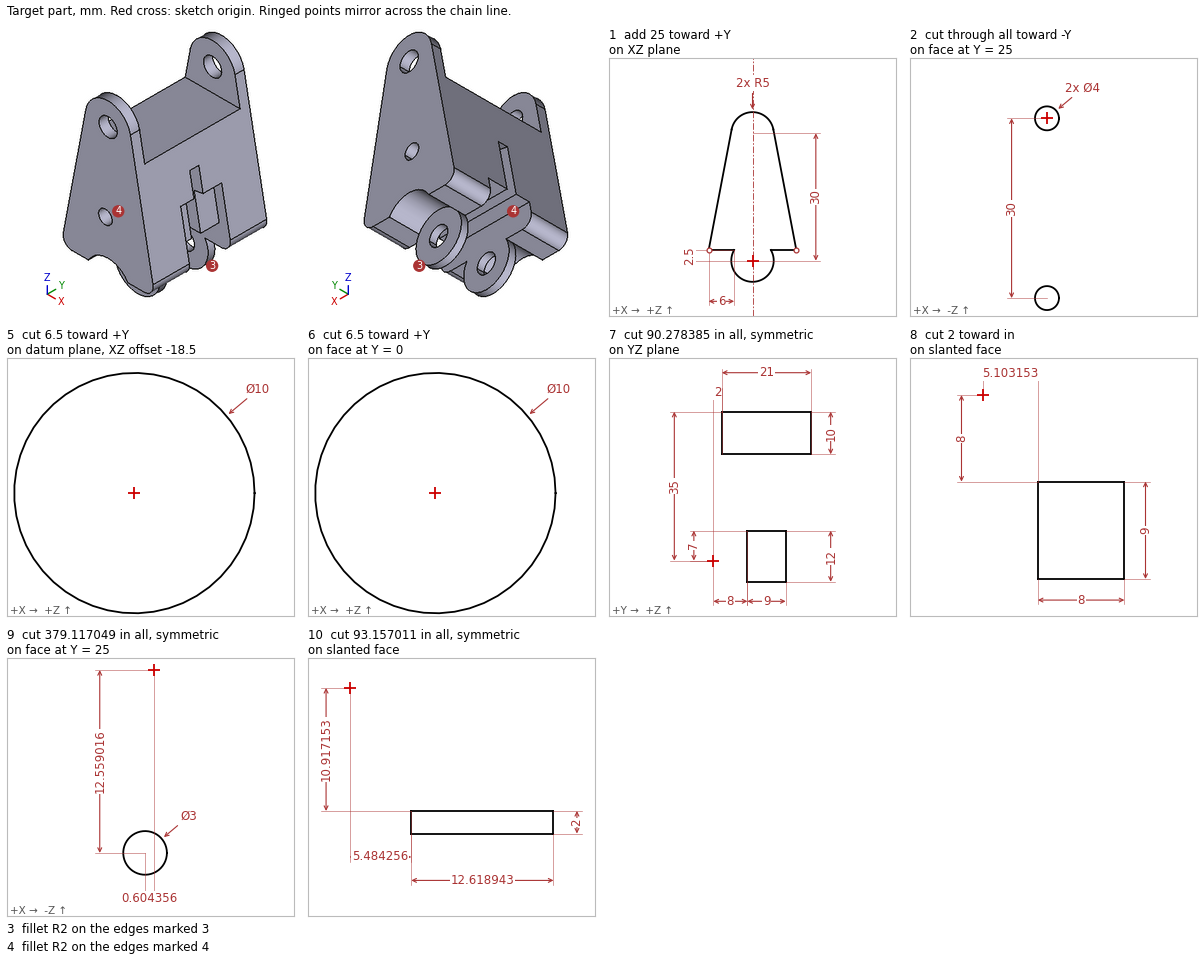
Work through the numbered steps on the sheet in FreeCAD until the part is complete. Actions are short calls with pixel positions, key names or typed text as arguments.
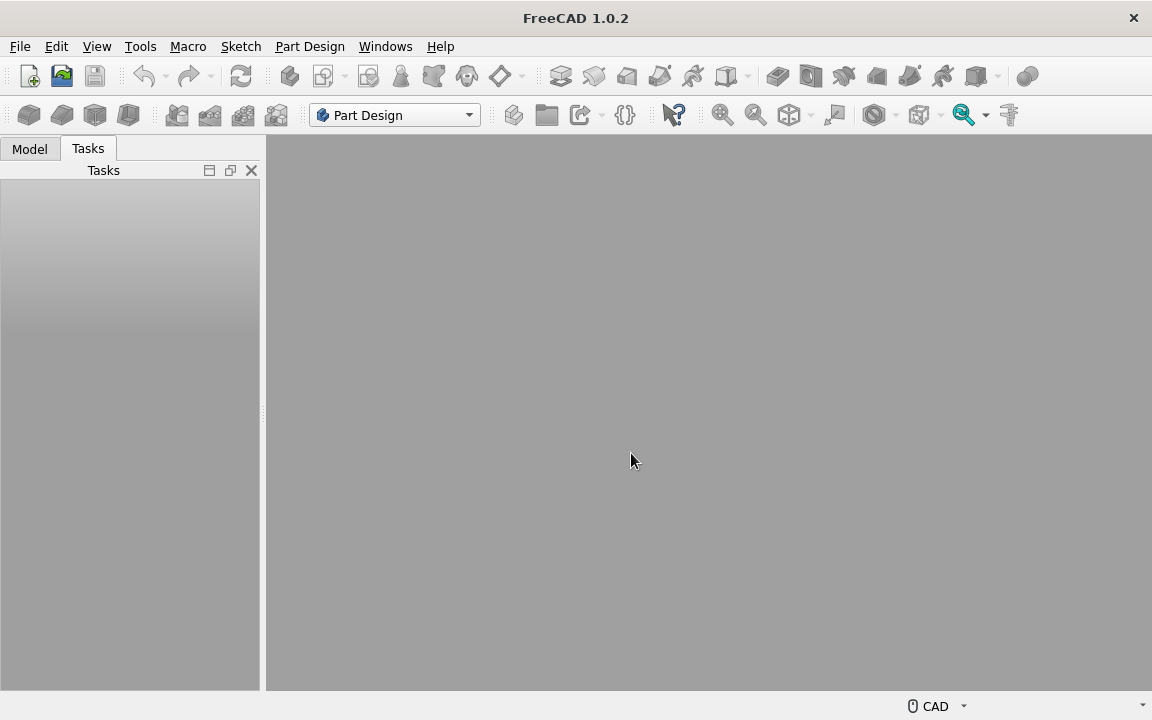
key(ctrl+n)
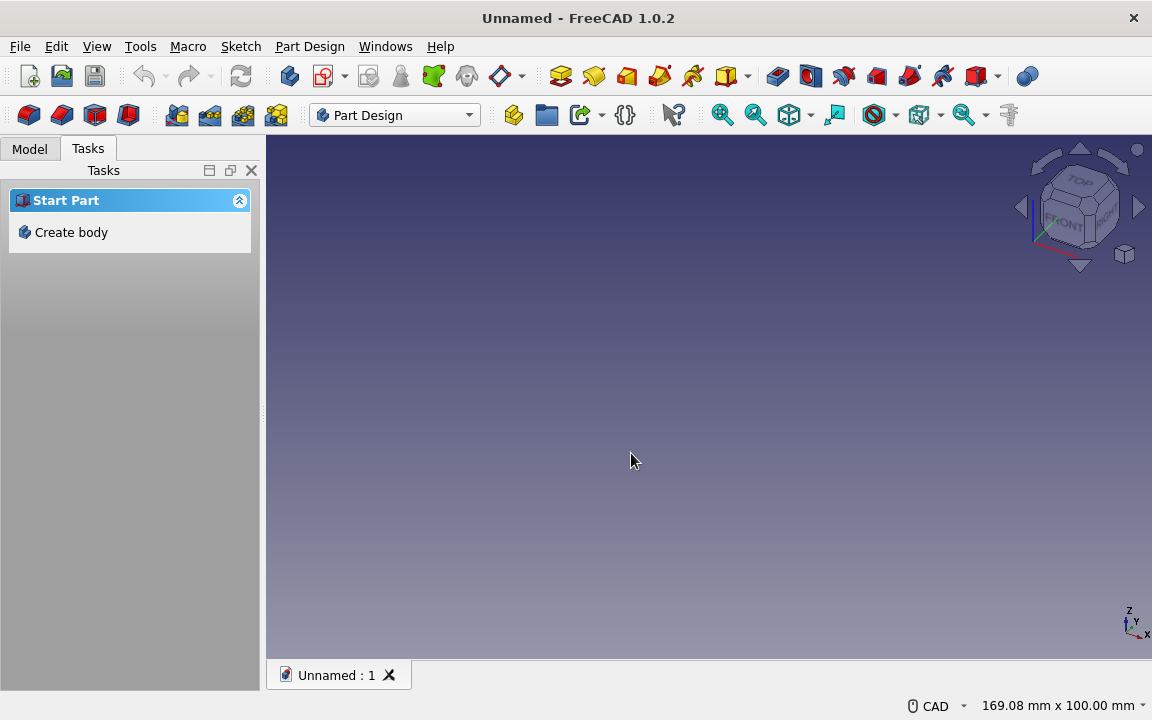
click(322, 76)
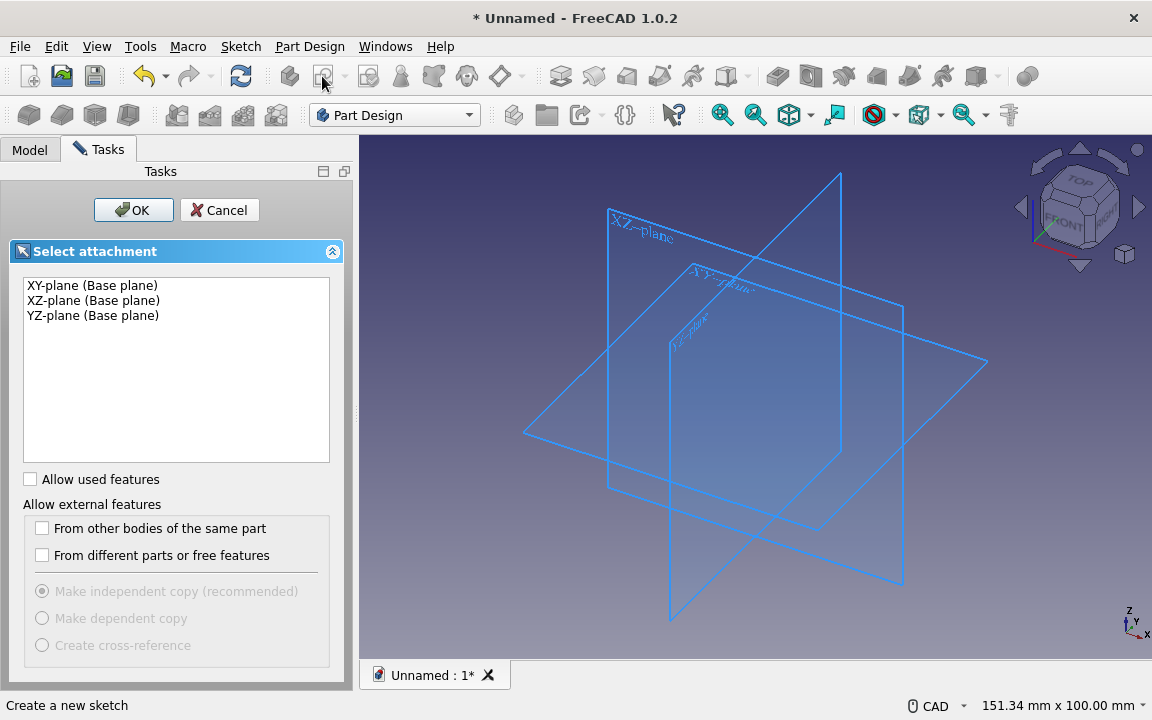
click(84, 300)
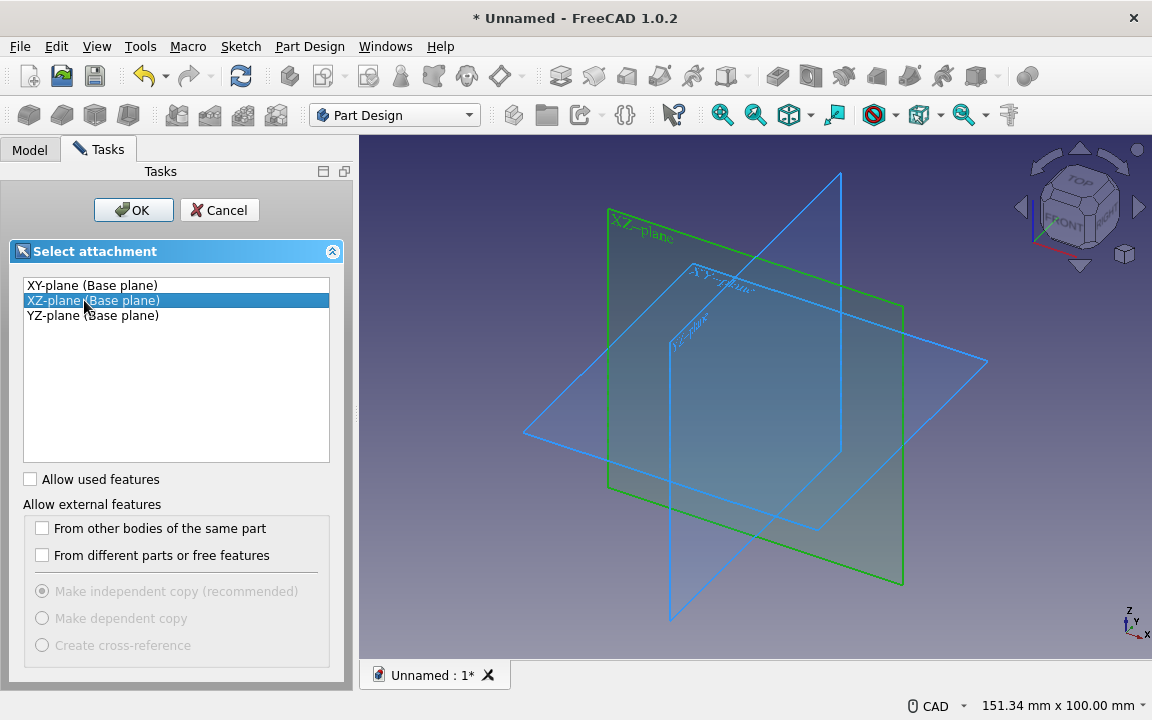
click(134, 210)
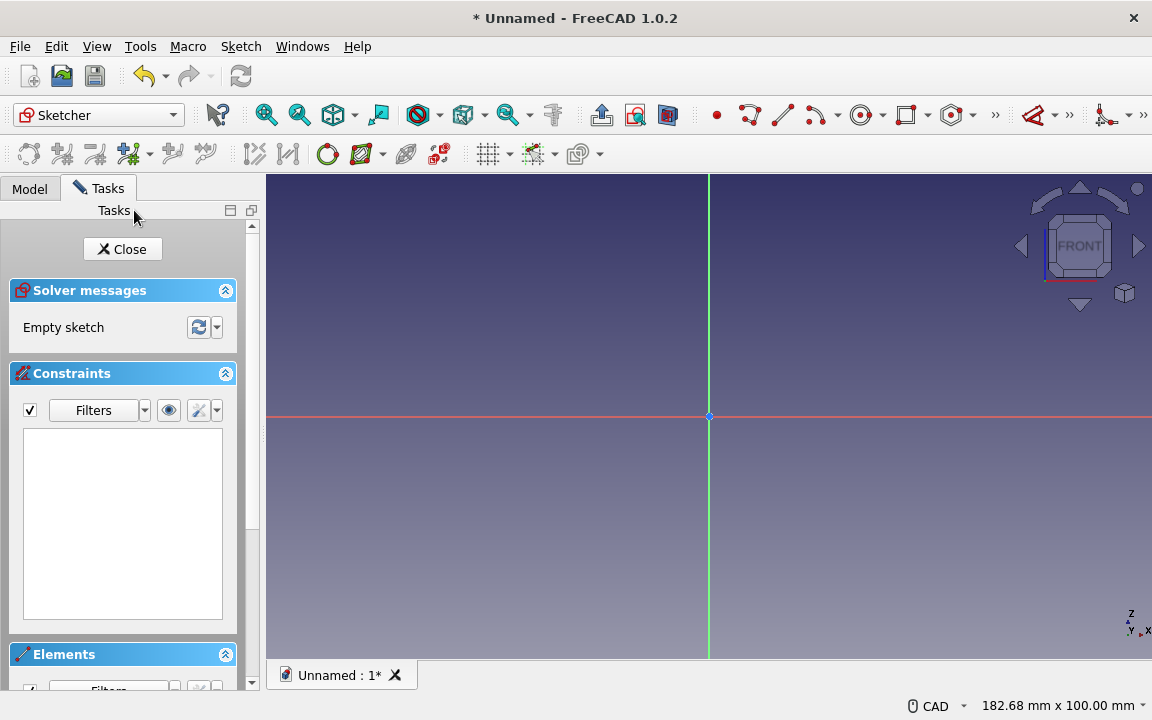
scroll(848, 202, up, 2)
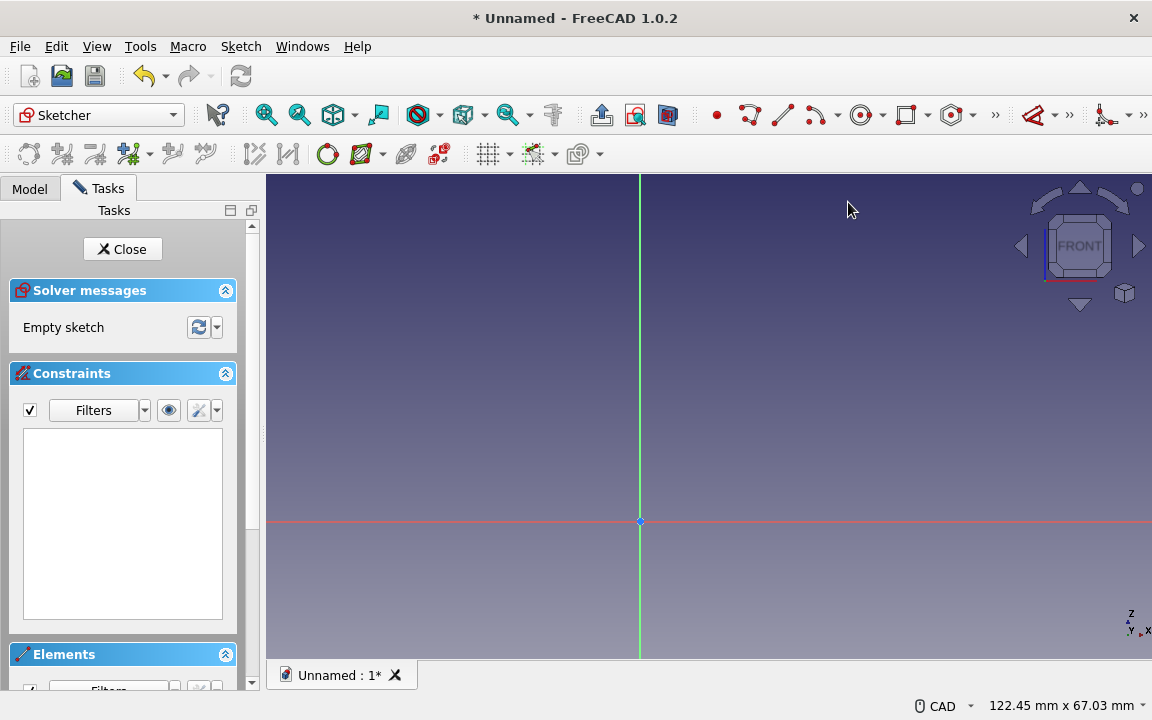
click(750, 116)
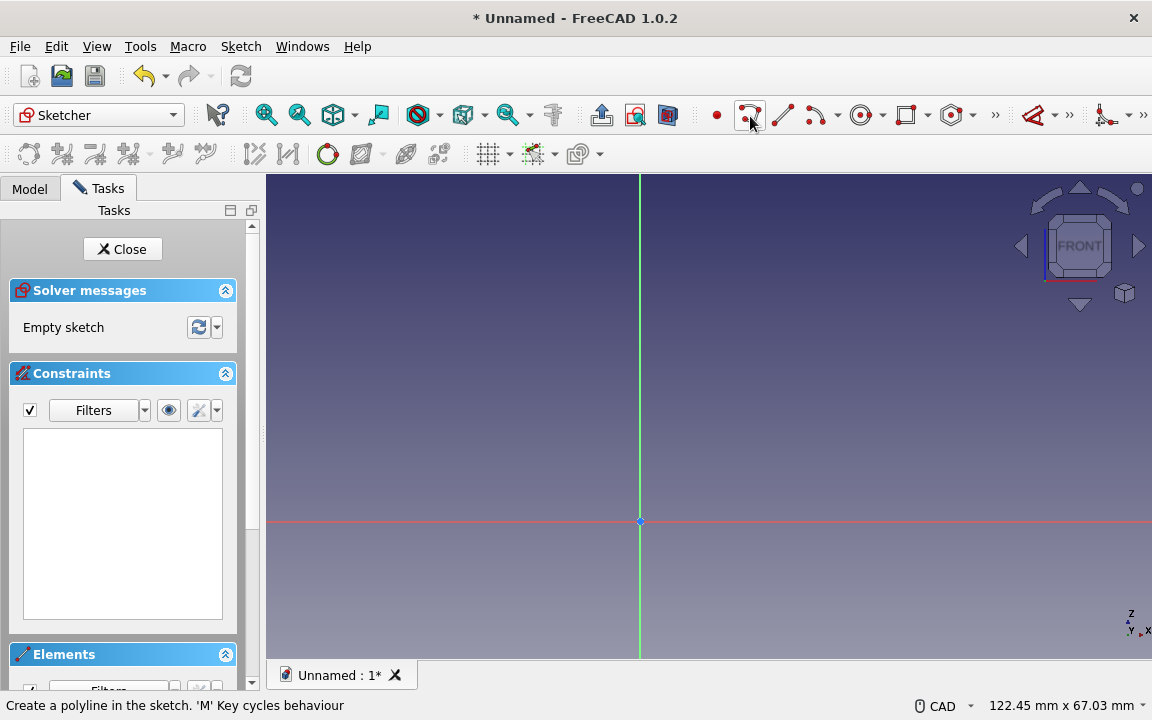
click(609, 504)
click(566, 504)
click(605, 298)
right_click(605, 298)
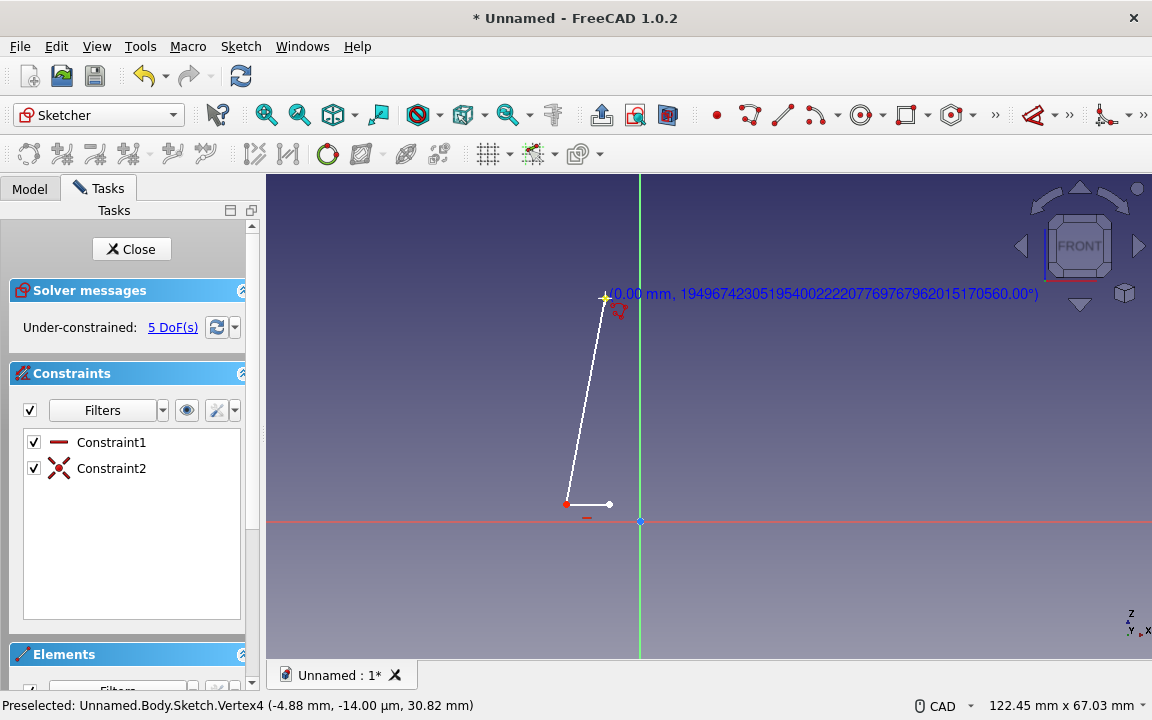
click(676, 298)
click(715, 504)
click(672, 504)
right_click(672, 504)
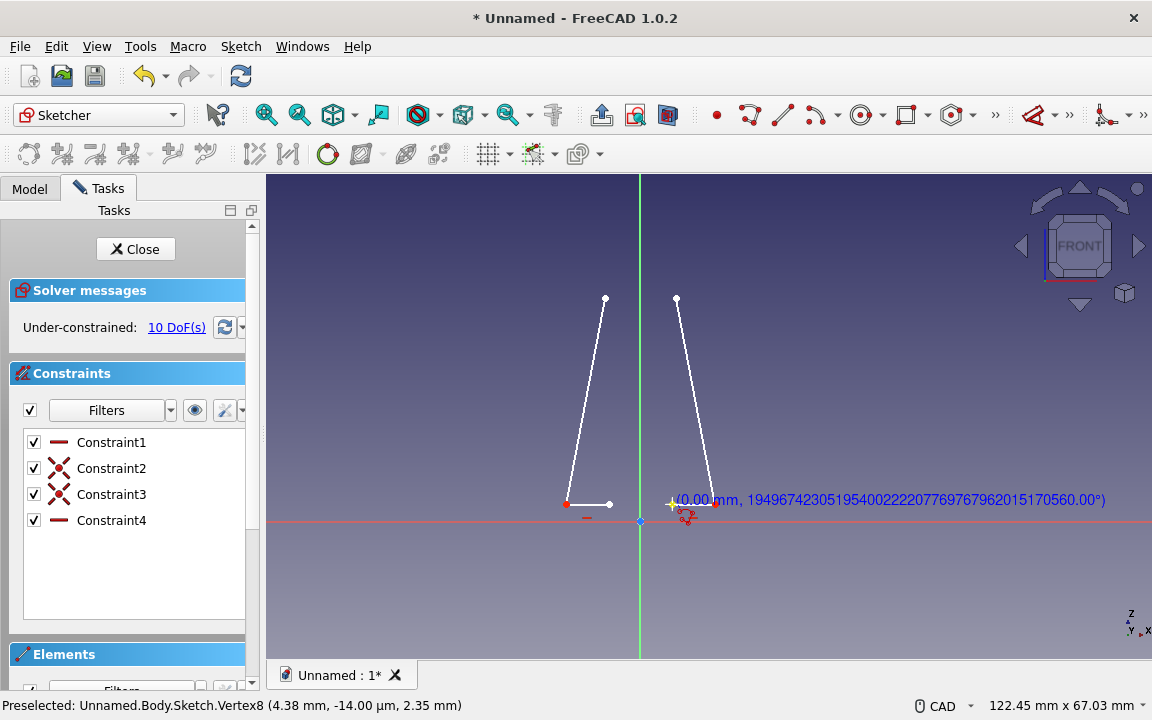
key(g)
key(3)
key(a)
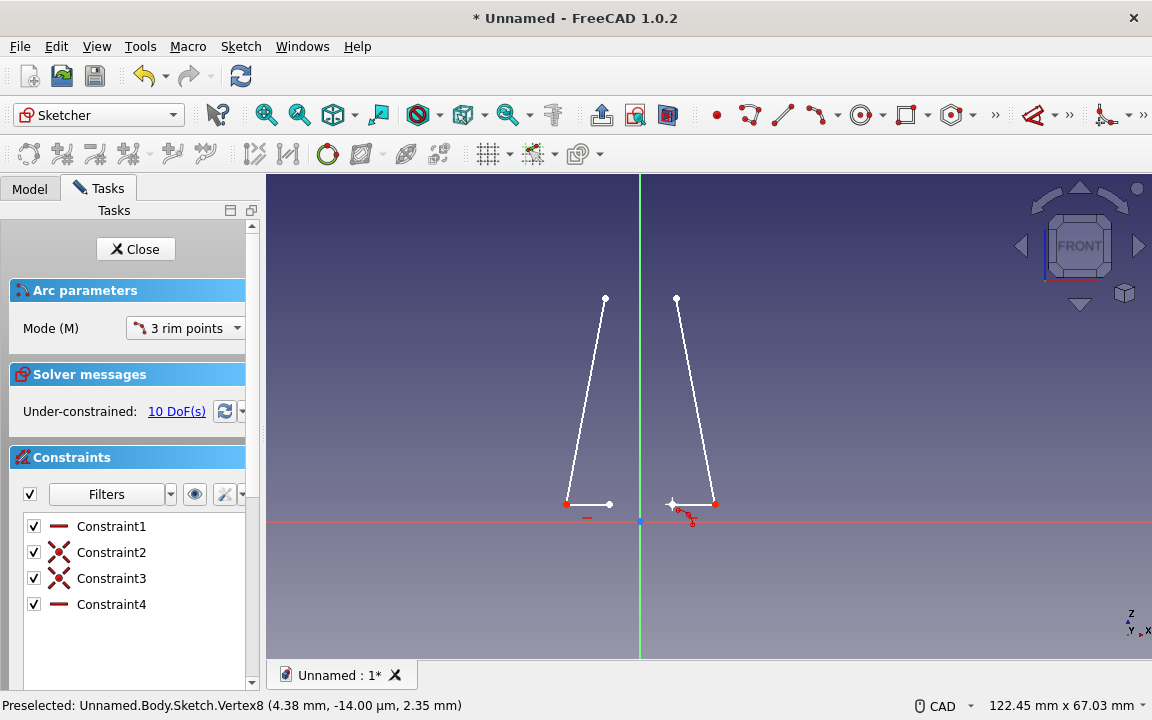
click(605, 299)
click(676, 299)
click(659, 274)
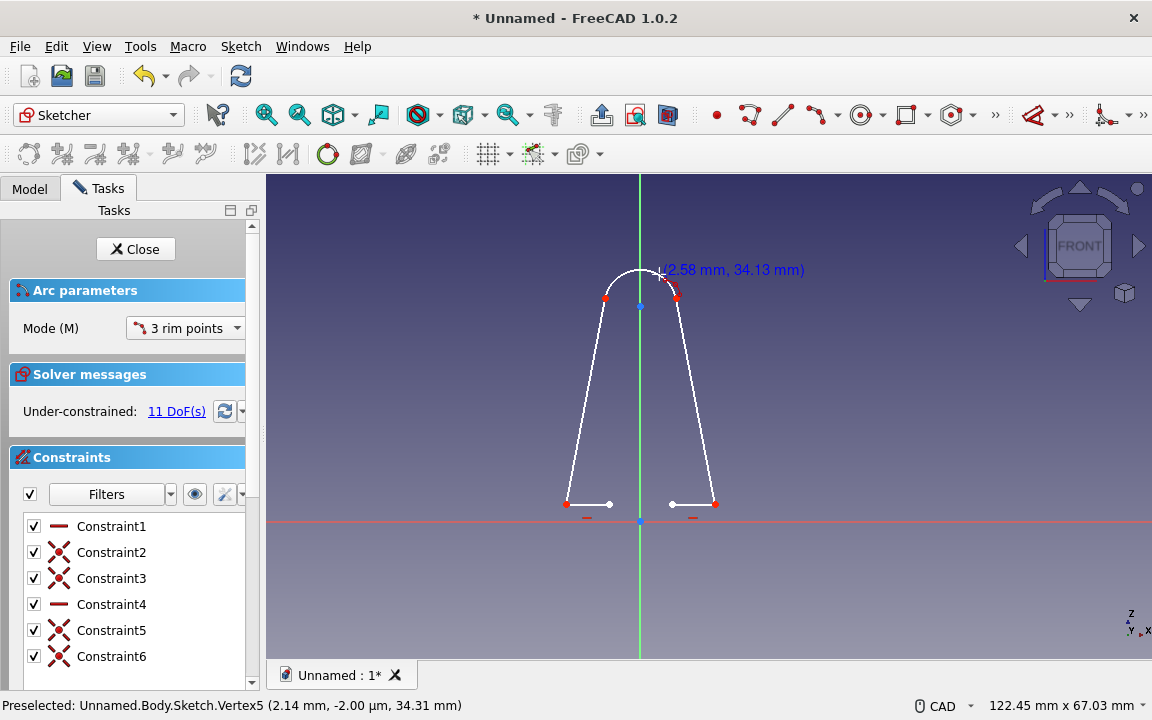
click(672, 505)
click(609, 505)
click(626, 555)
key(Escape)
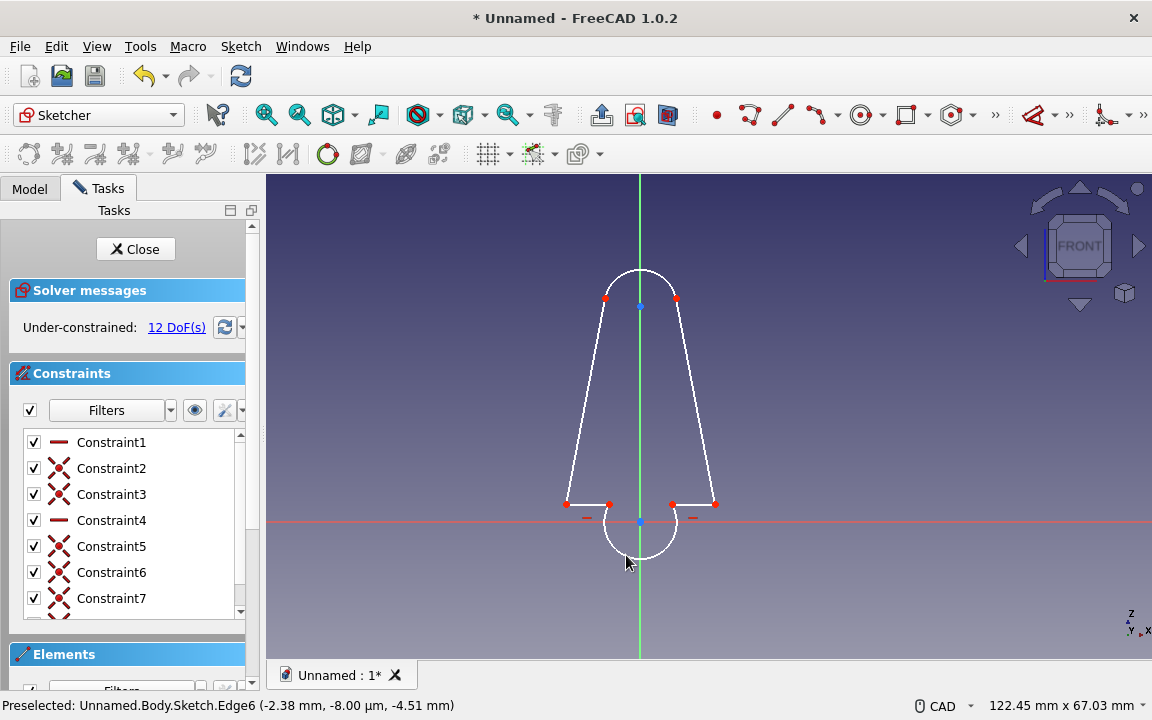
click(578, 443)